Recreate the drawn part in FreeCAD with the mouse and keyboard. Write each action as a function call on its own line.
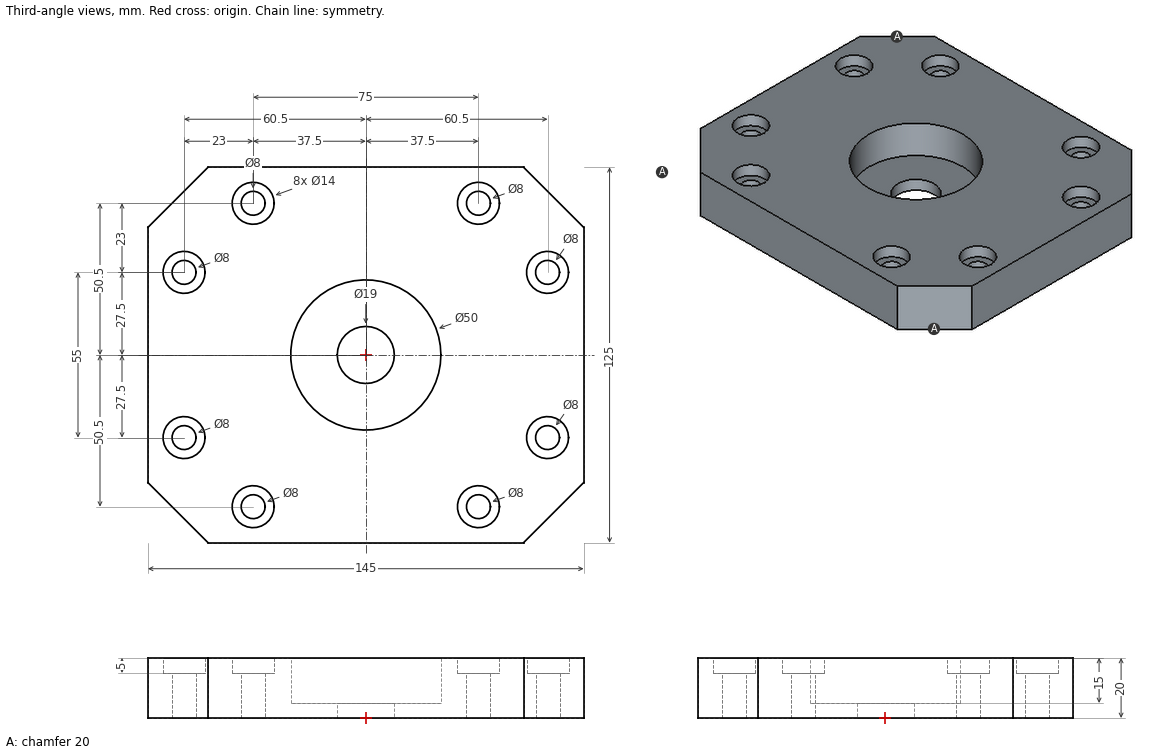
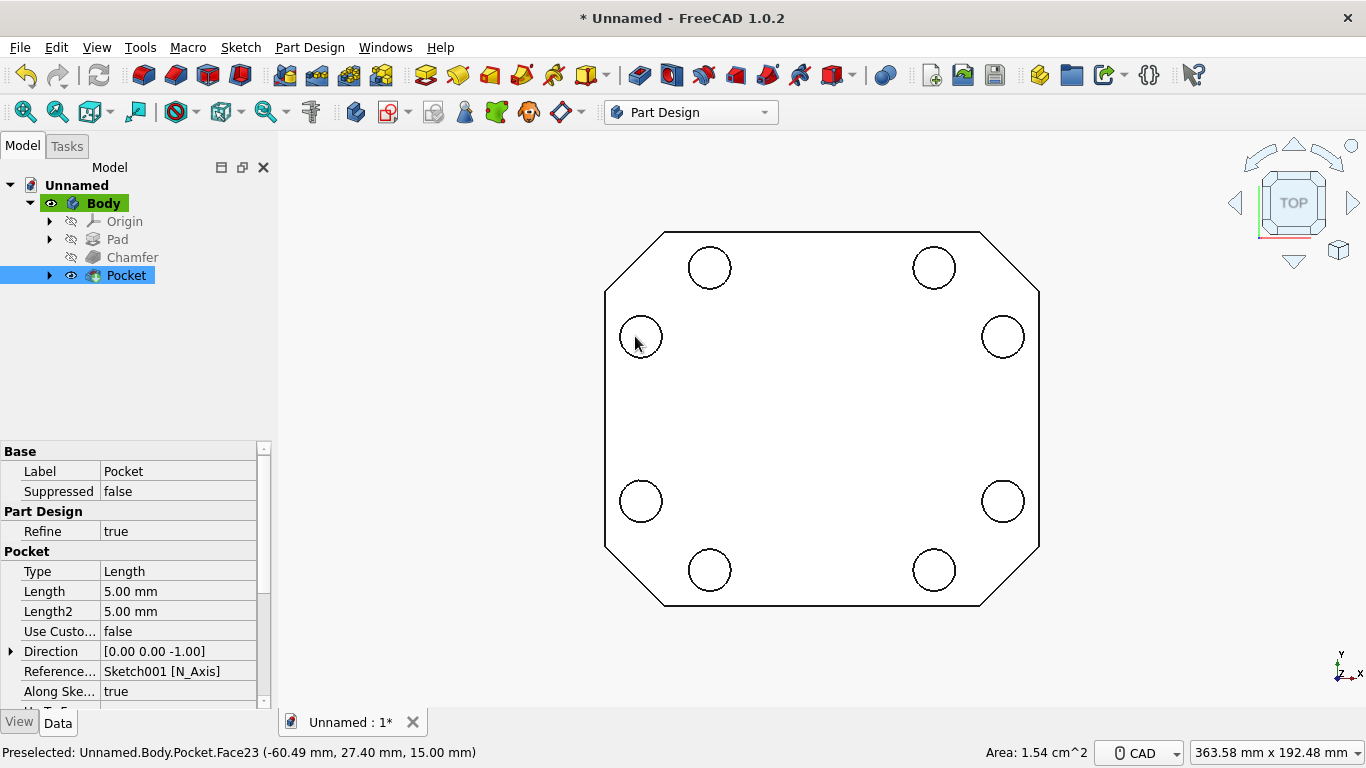
click(388, 112)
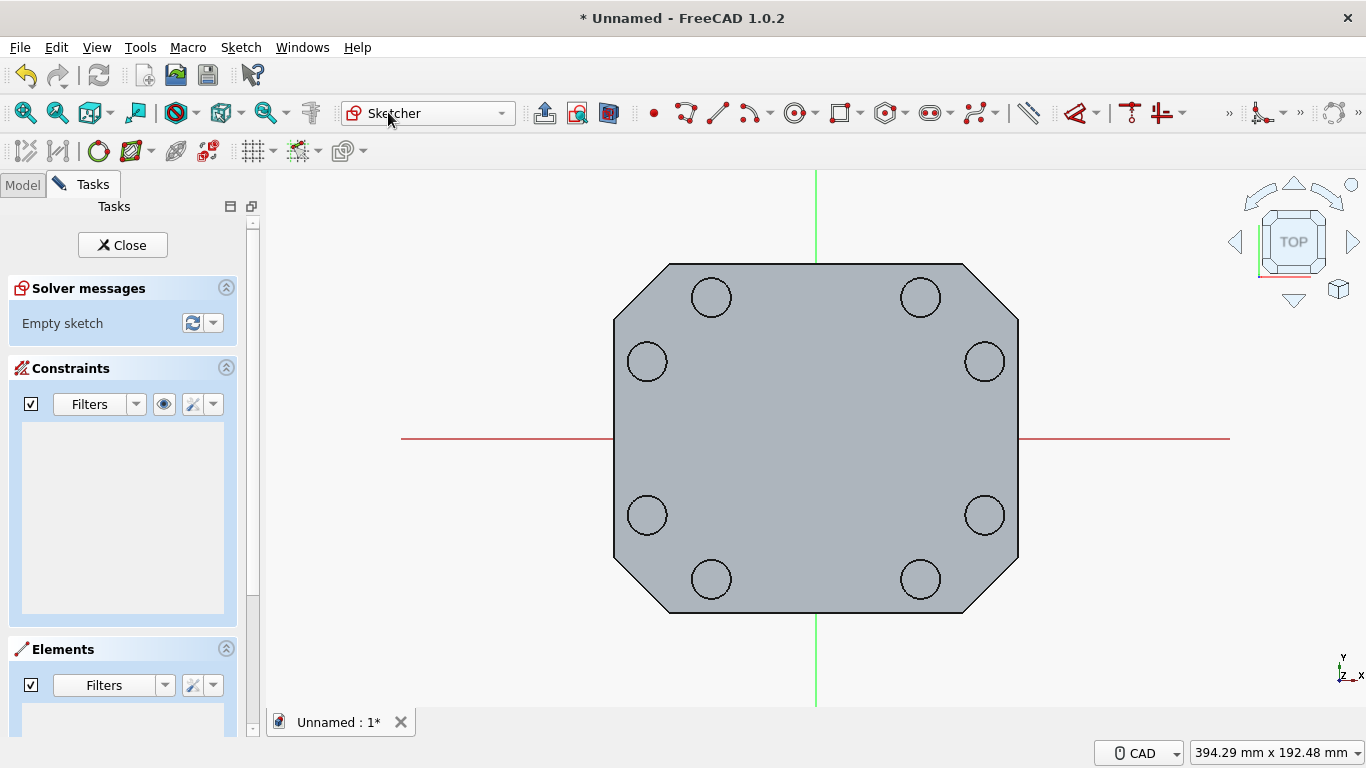
click(610, 114)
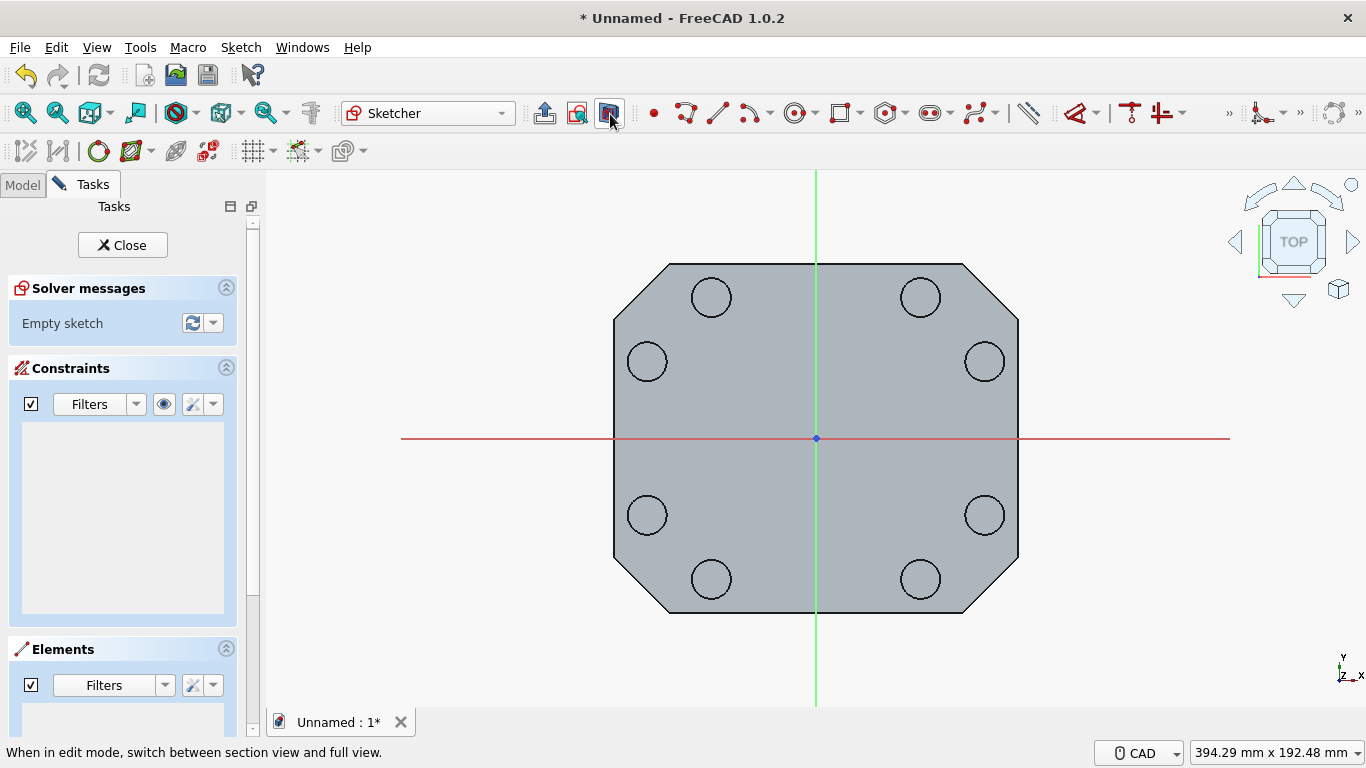
scroll(709, 288, up, 14)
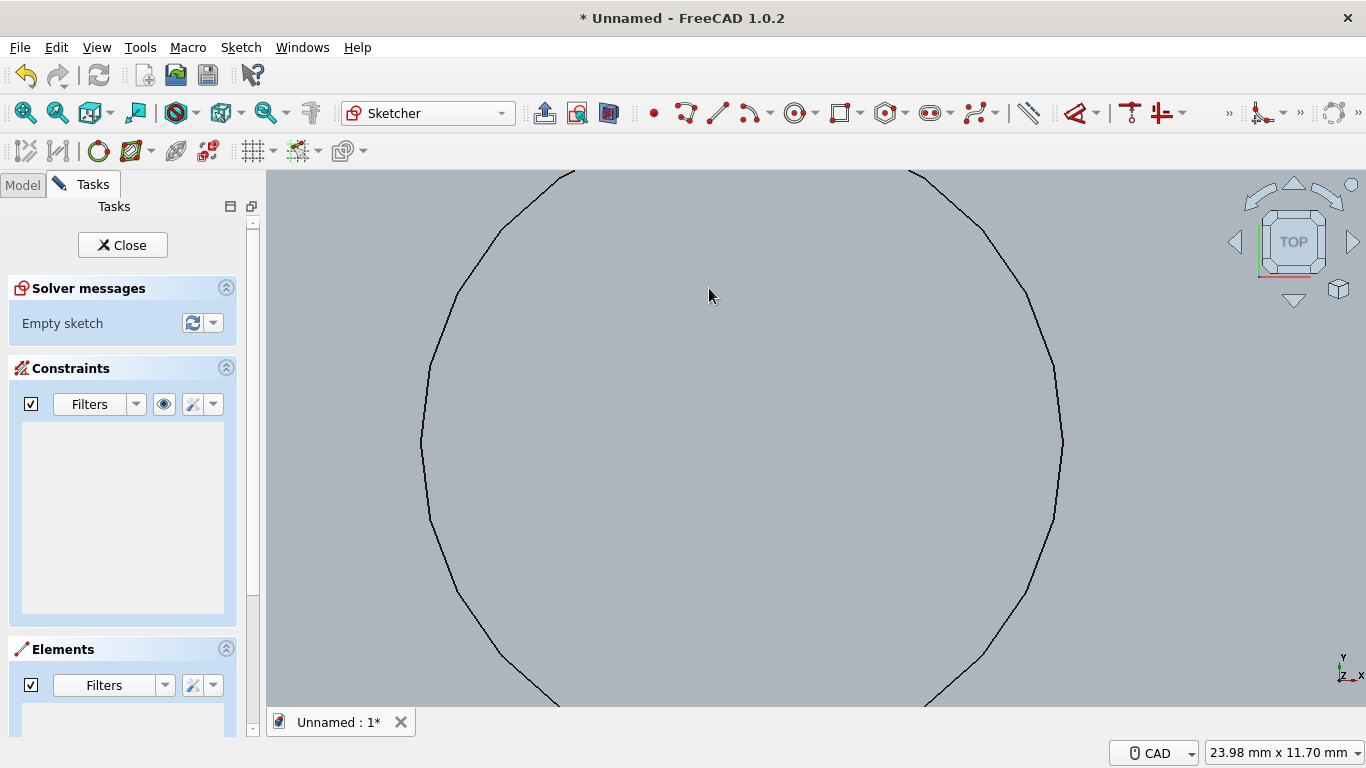
click(796, 114)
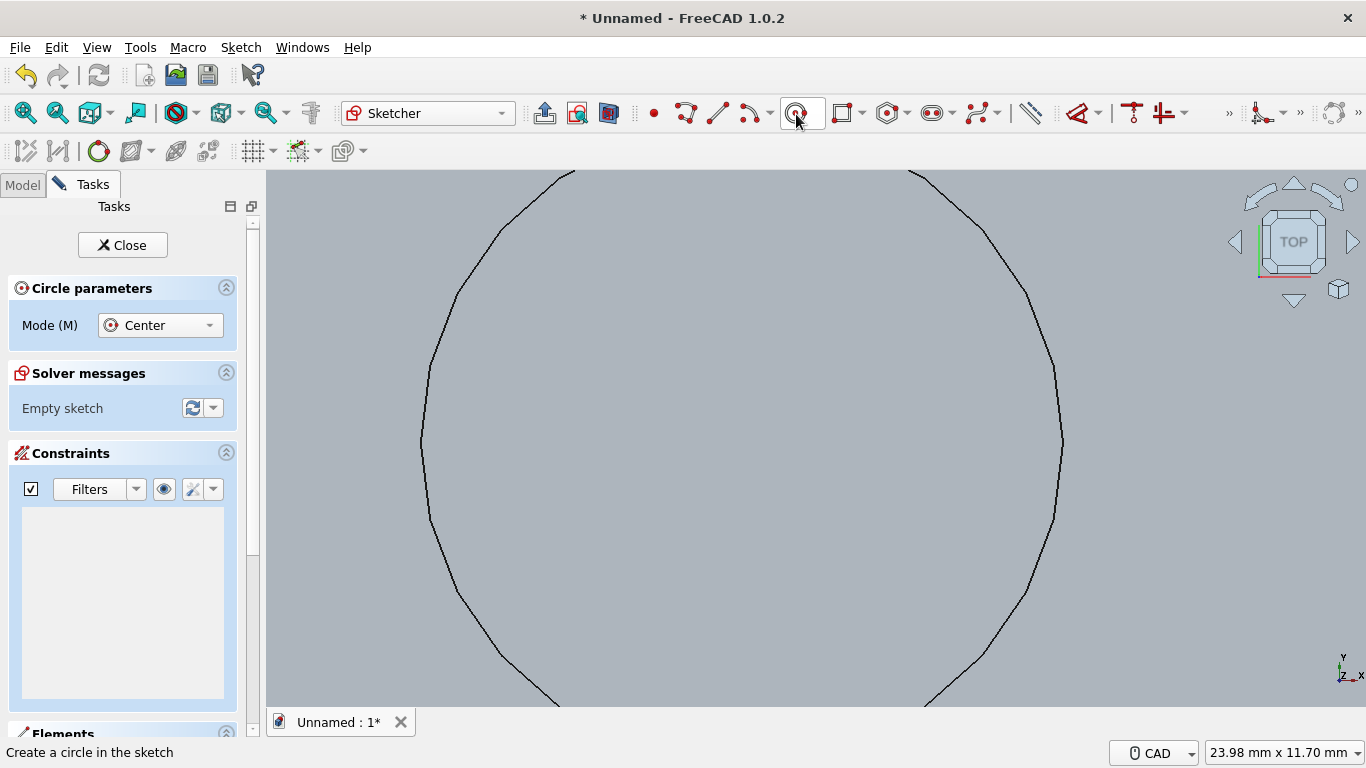
click(742, 443)
click(872, 313)
key(Escape)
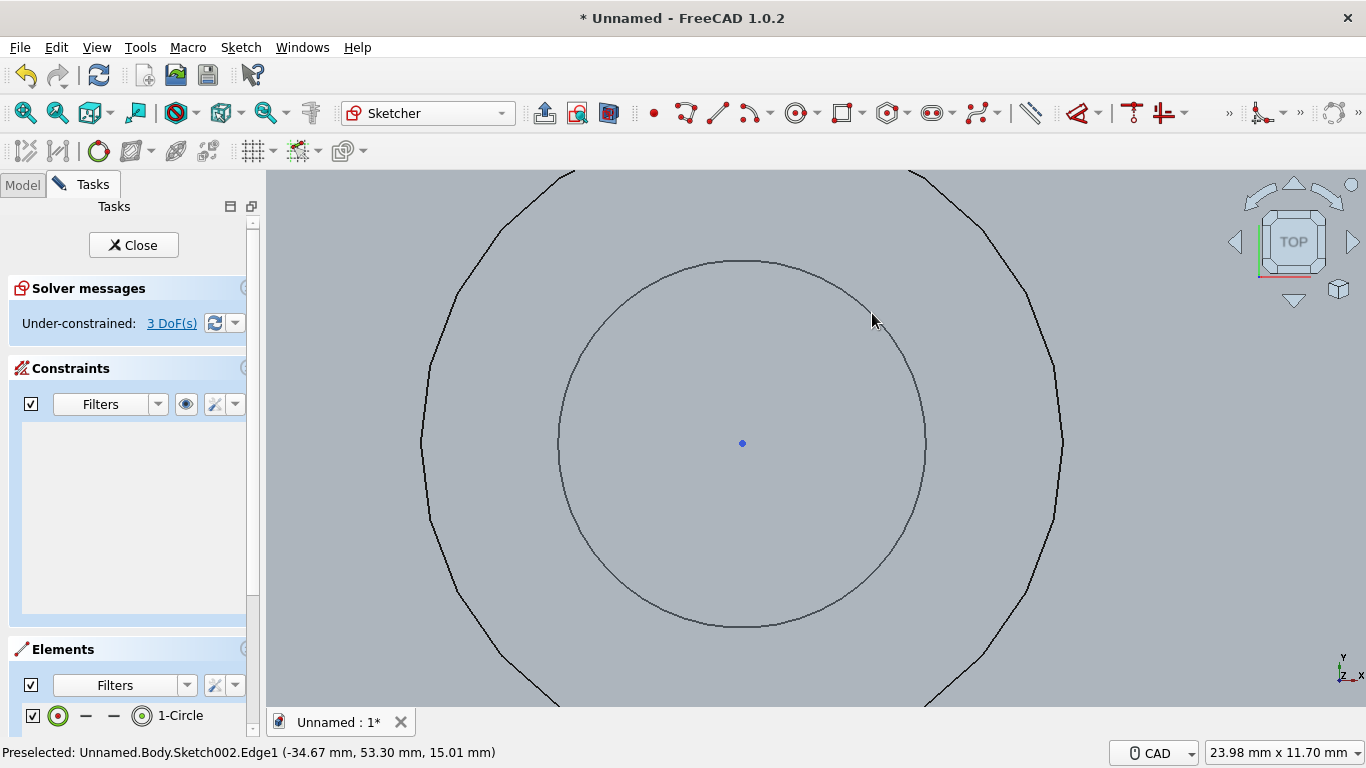
click(1078, 114)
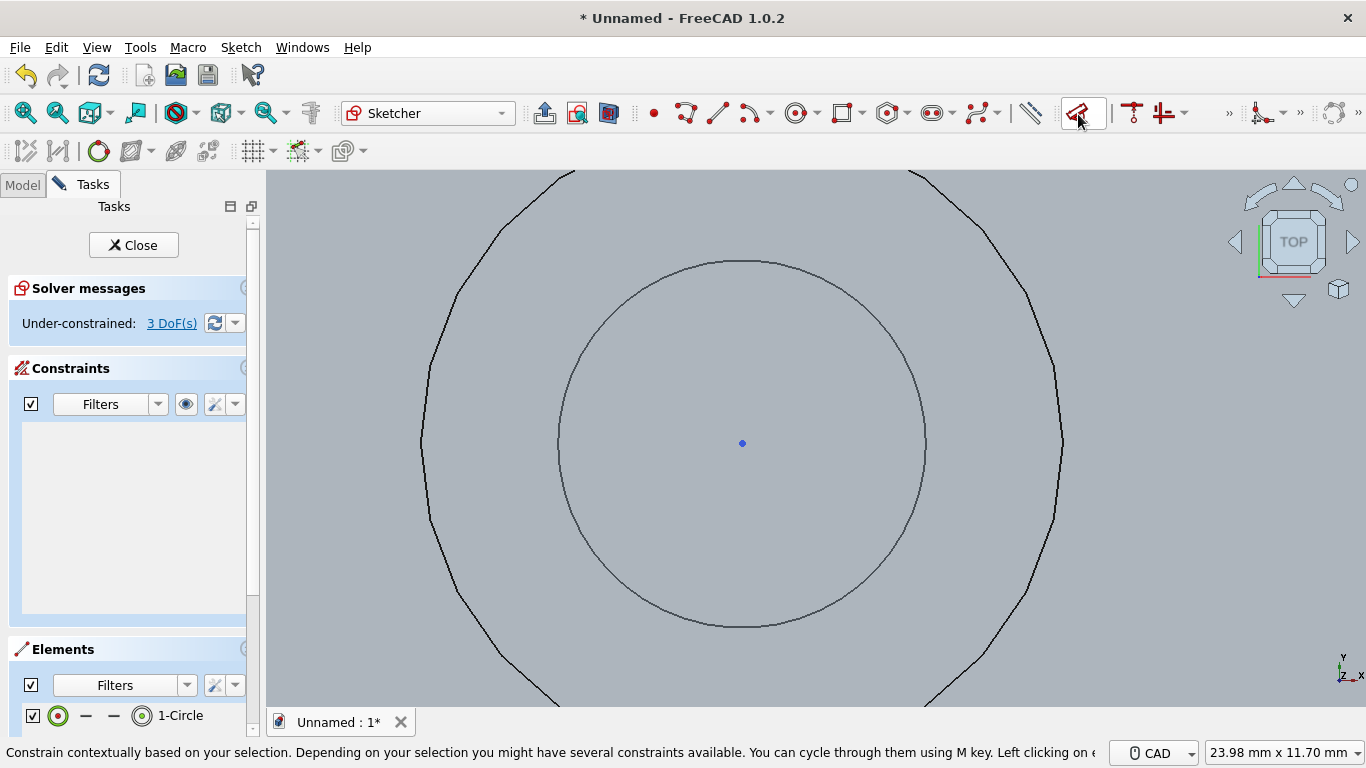
click(872, 314)
click(895, 291)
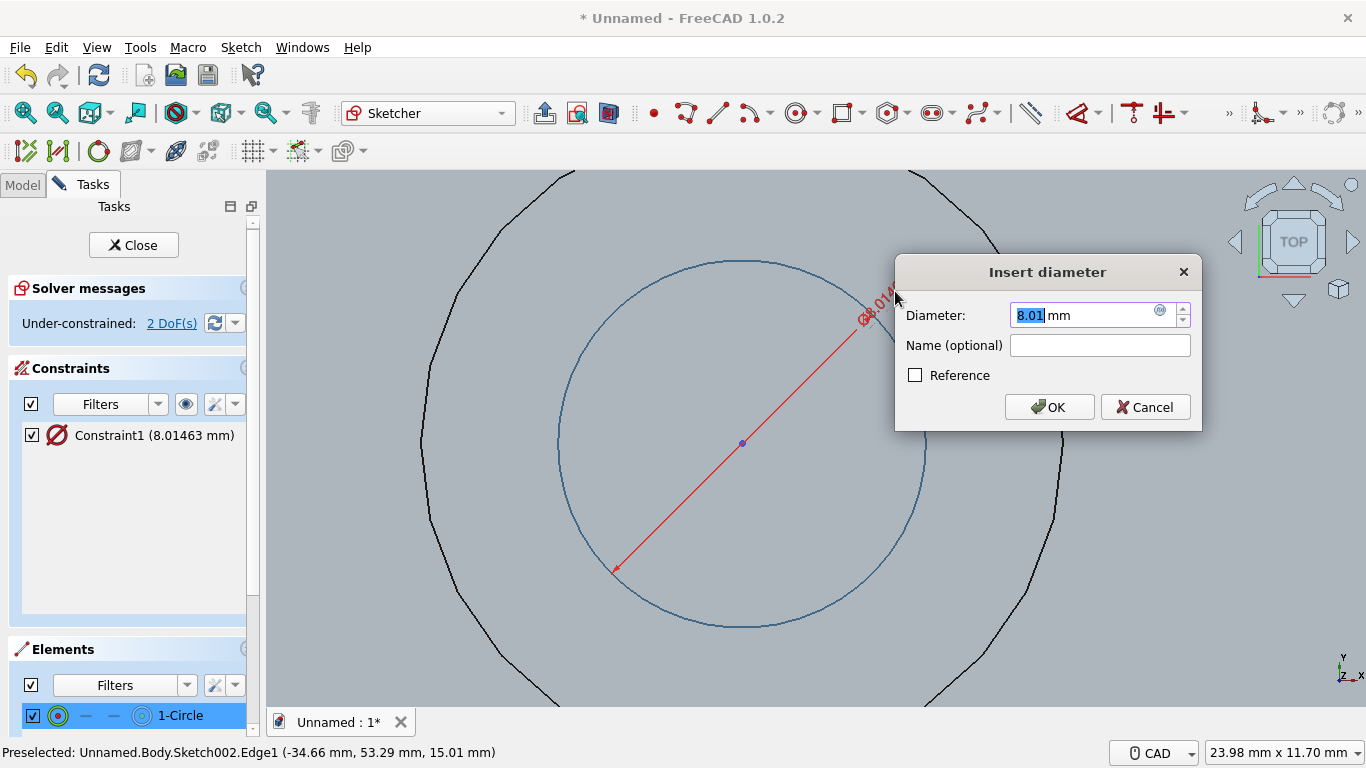
text(8)
key(Return)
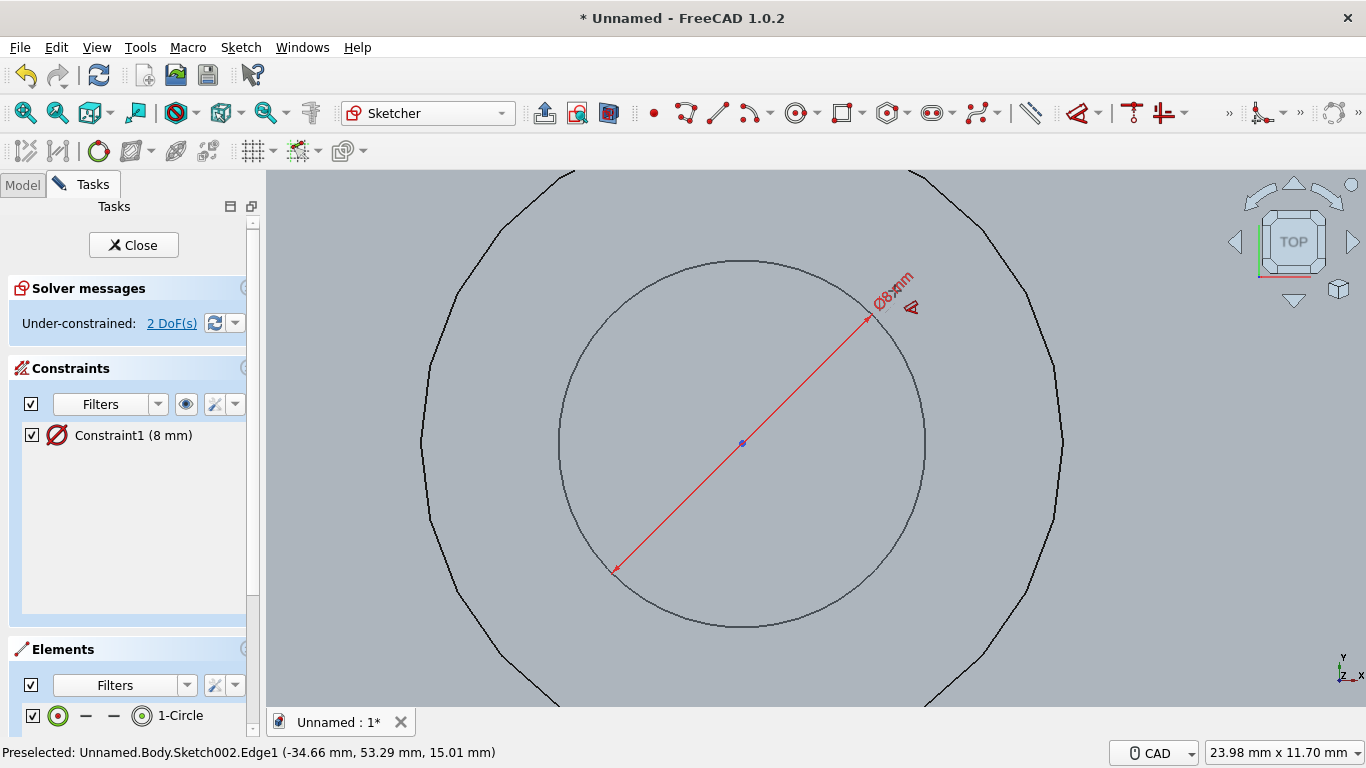
click(742, 444)
click(972, 410)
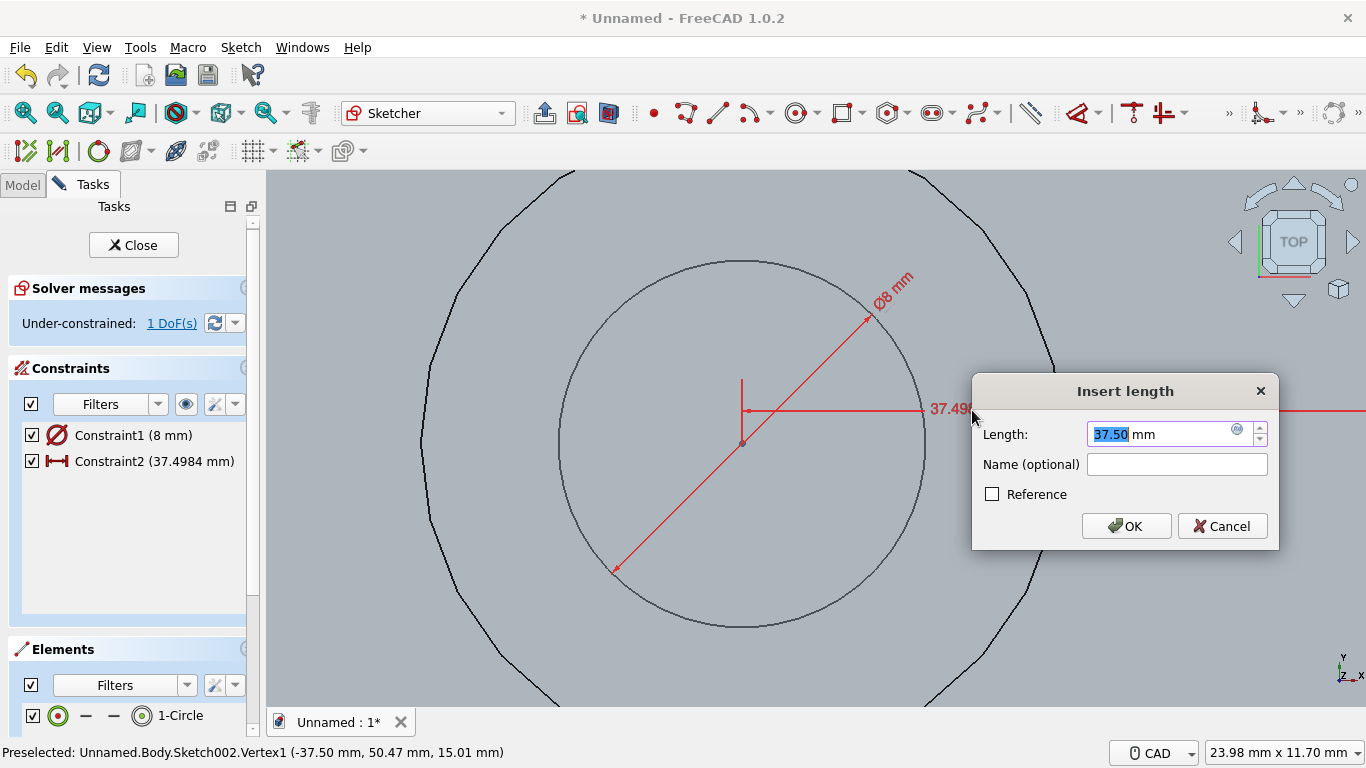
text(37.5)
key(Return)